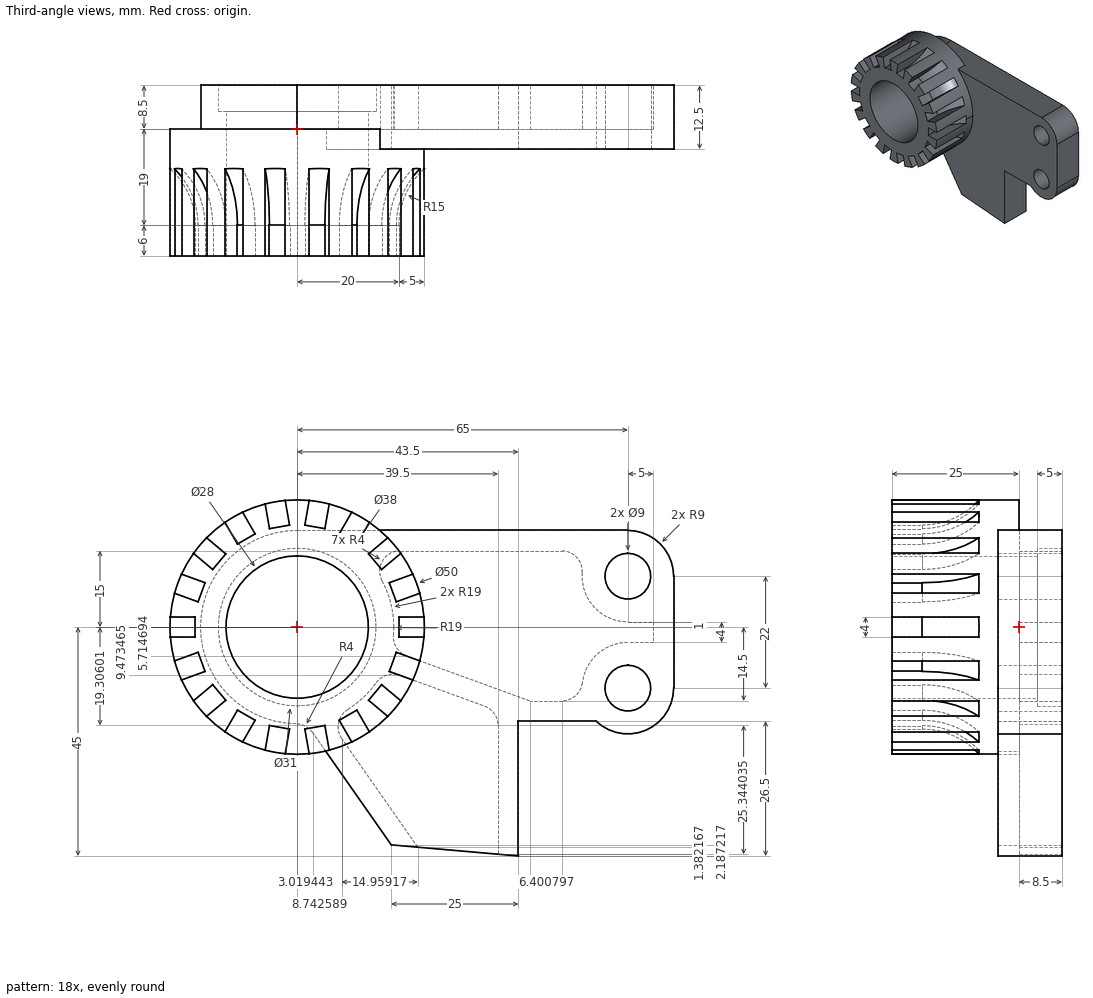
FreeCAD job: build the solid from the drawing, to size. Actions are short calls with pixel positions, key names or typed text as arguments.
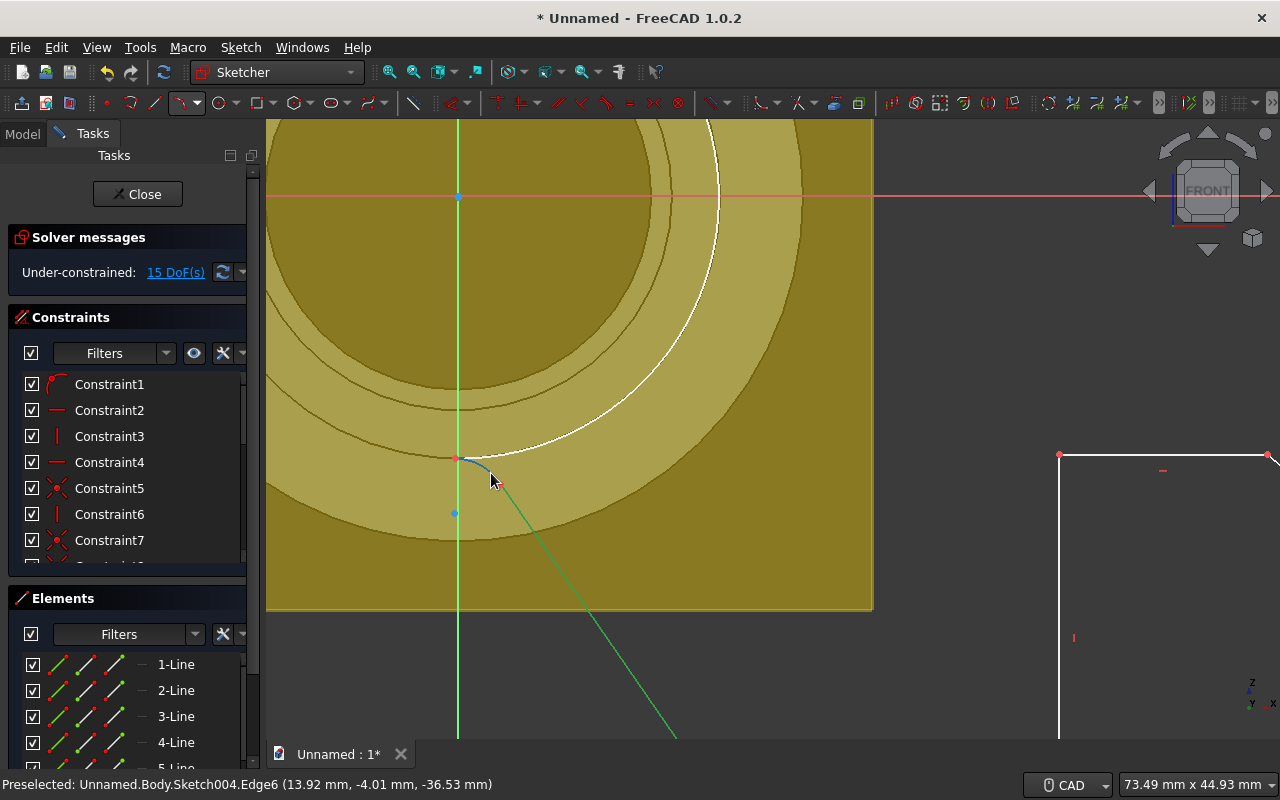
click(490, 472)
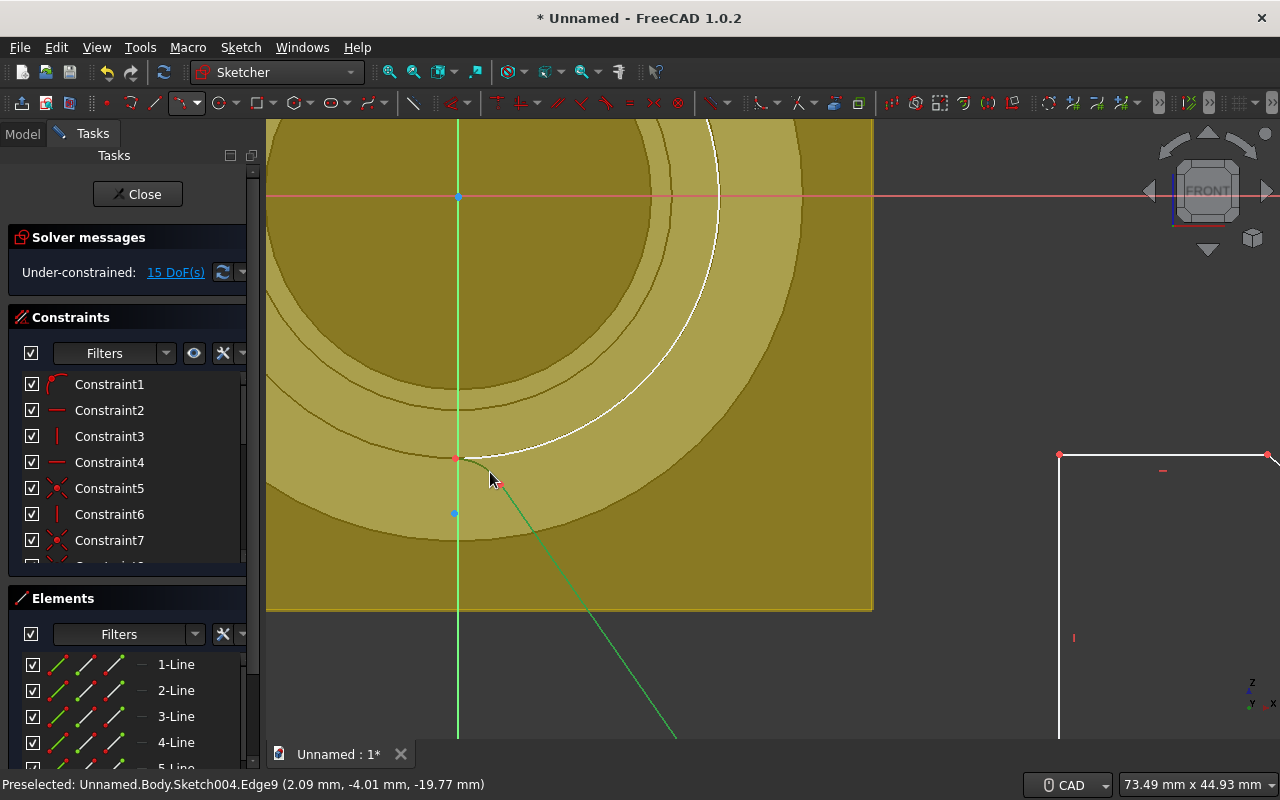
click(606, 104)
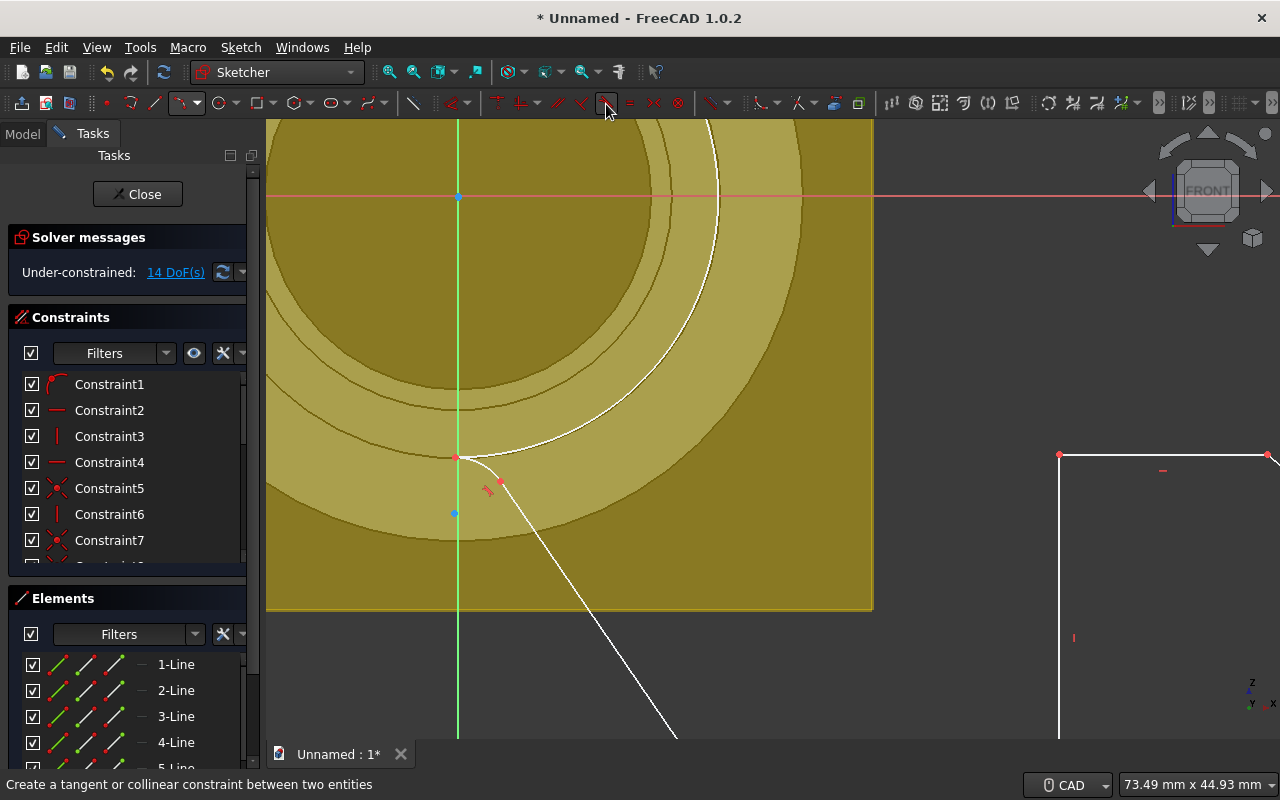
click(490, 470)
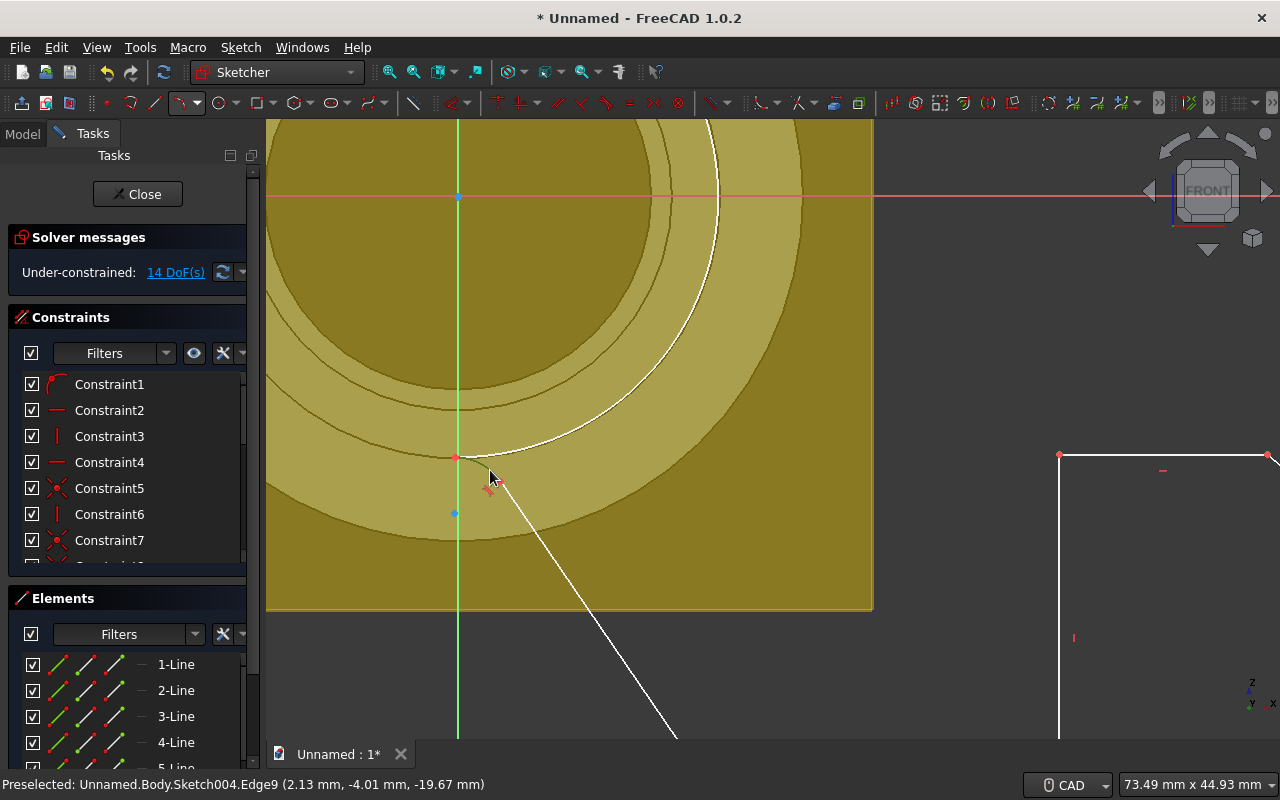
click(667, 352)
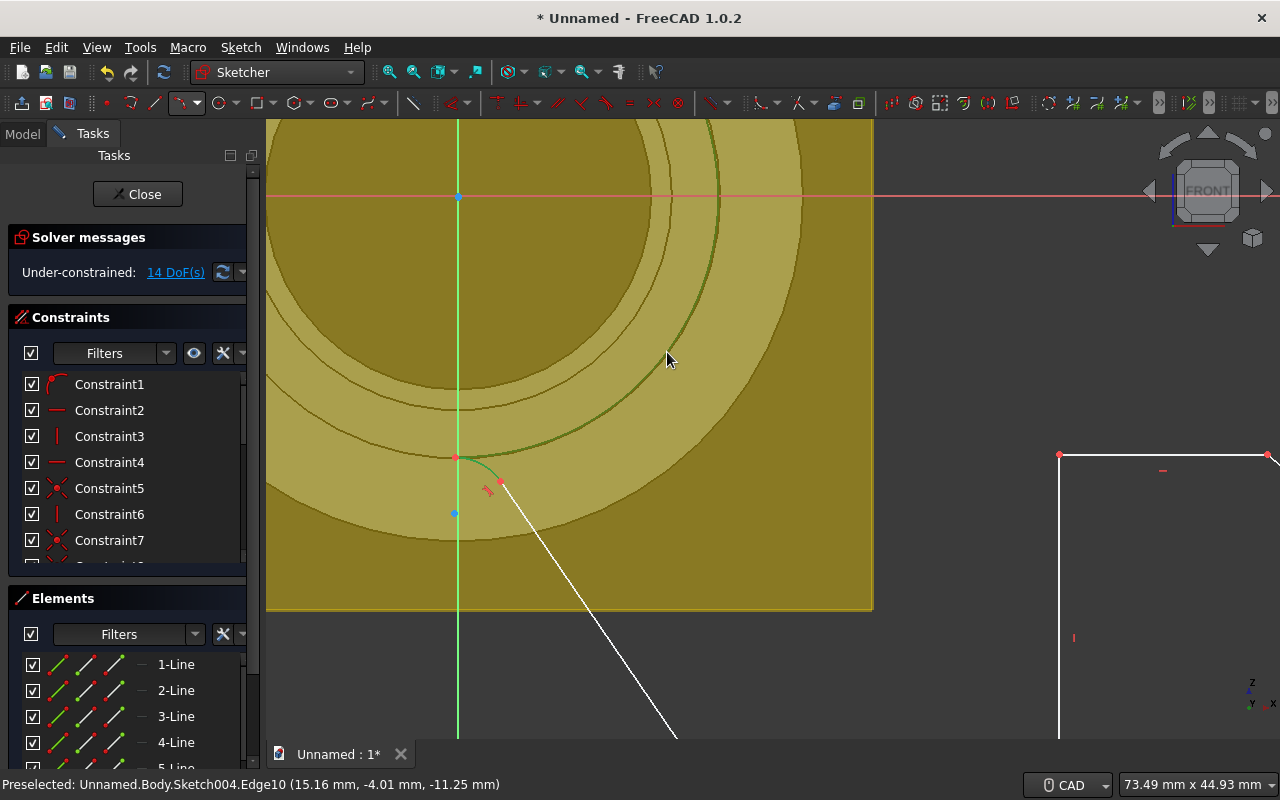
click(606, 104)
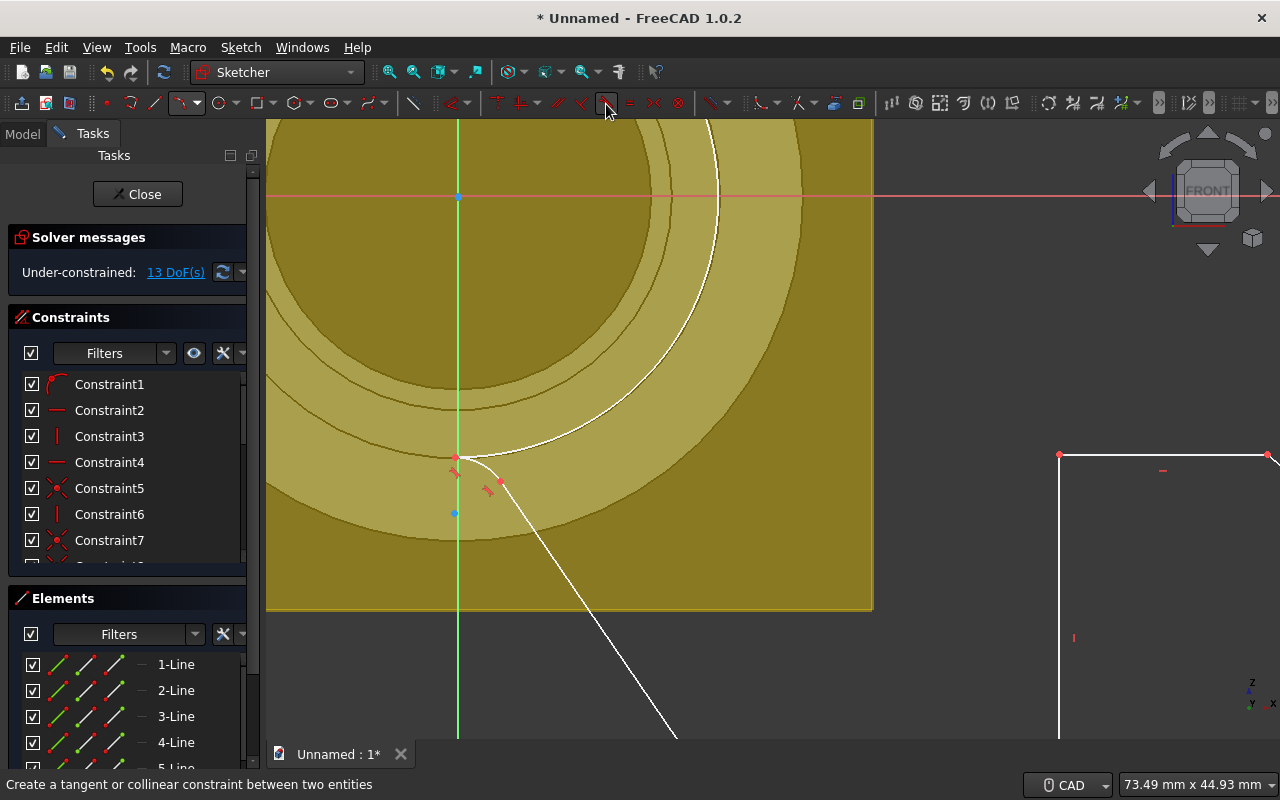
scroll(490, 472, down, 4)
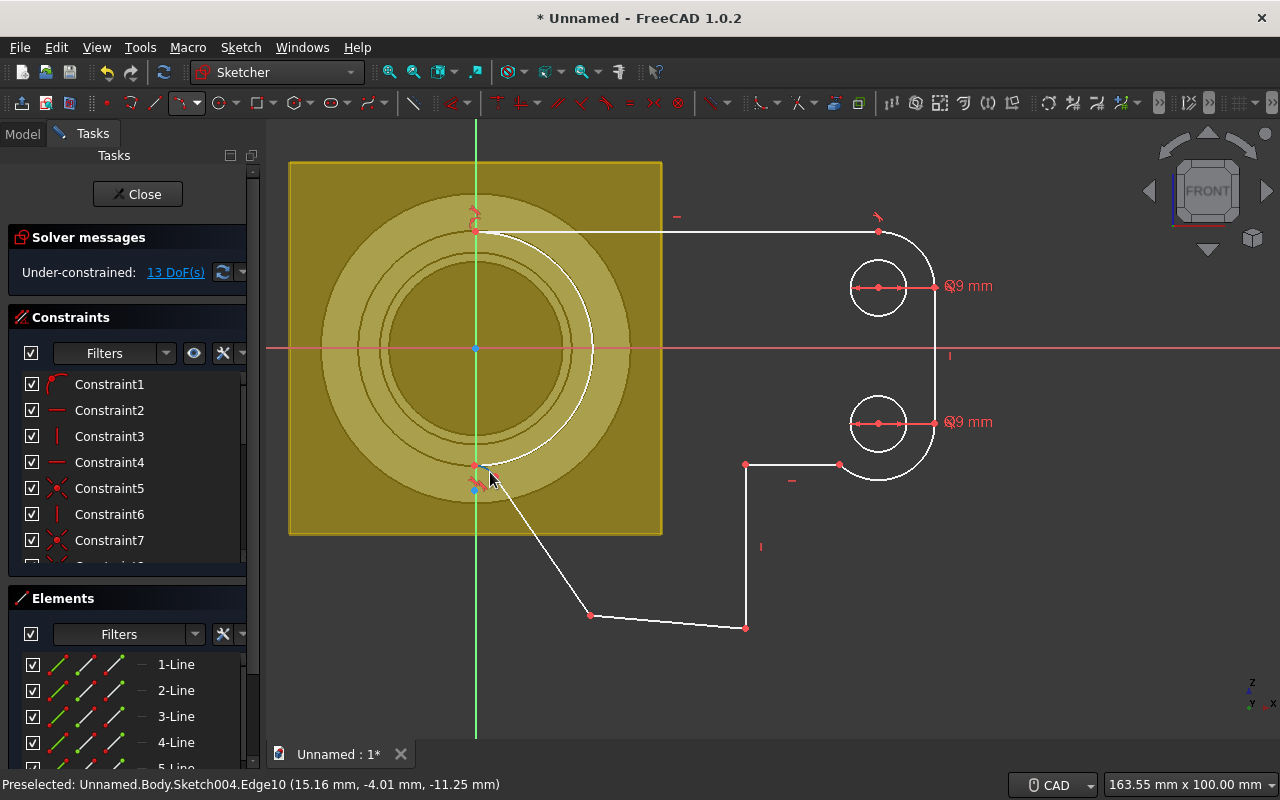
click(928, 263)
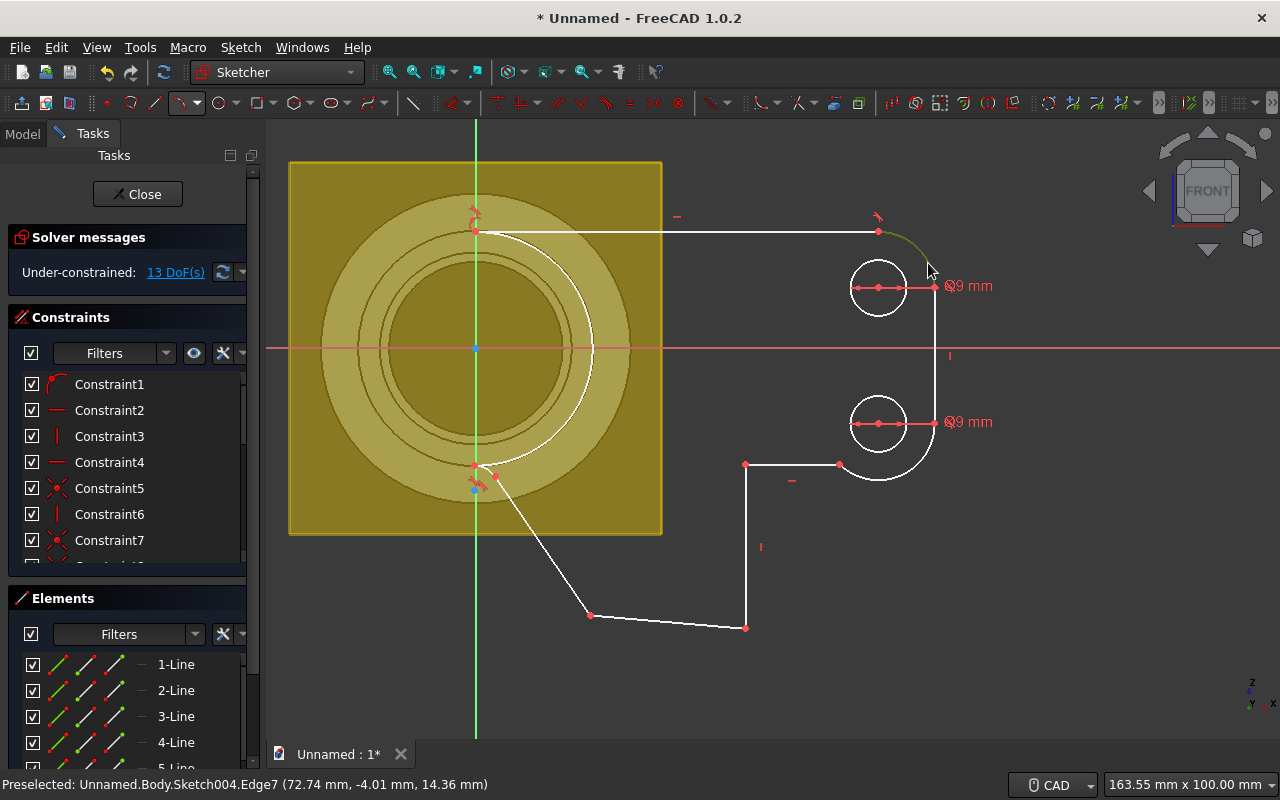
click(875, 480)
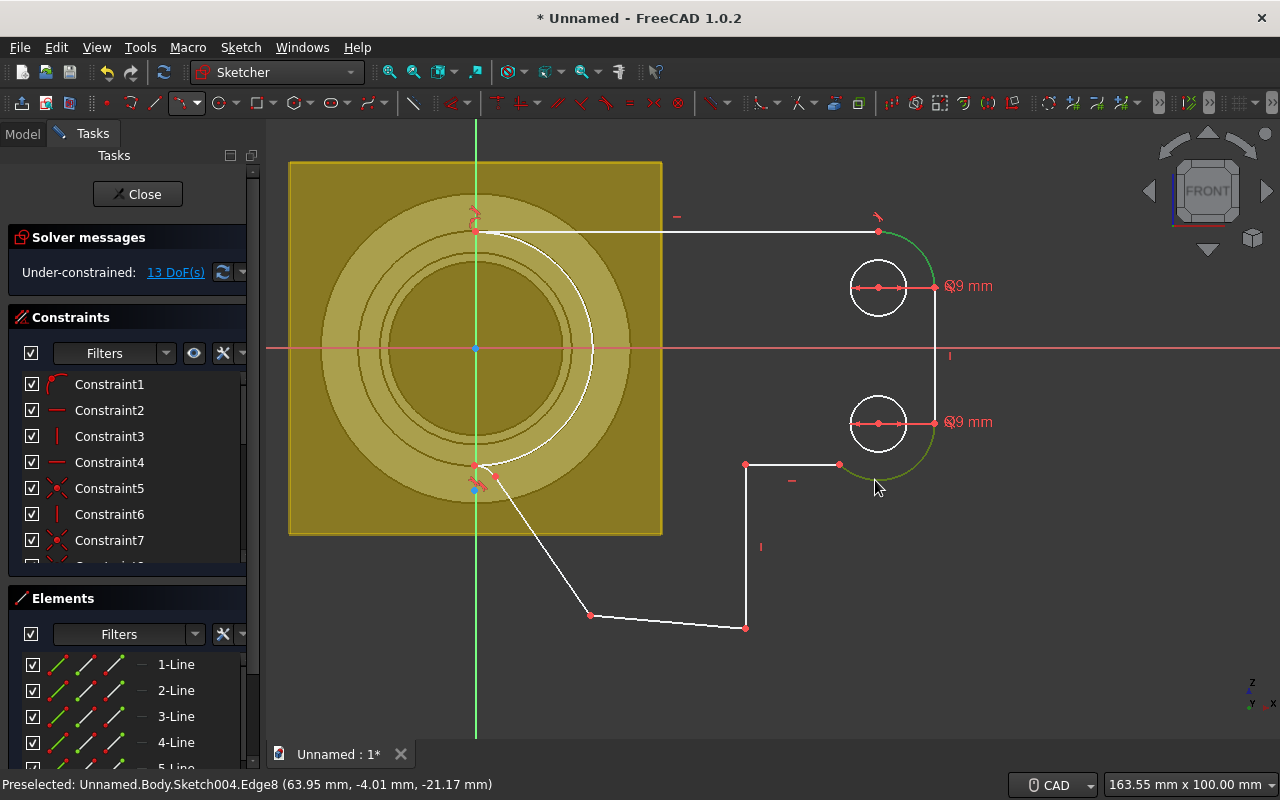
click(630, 104)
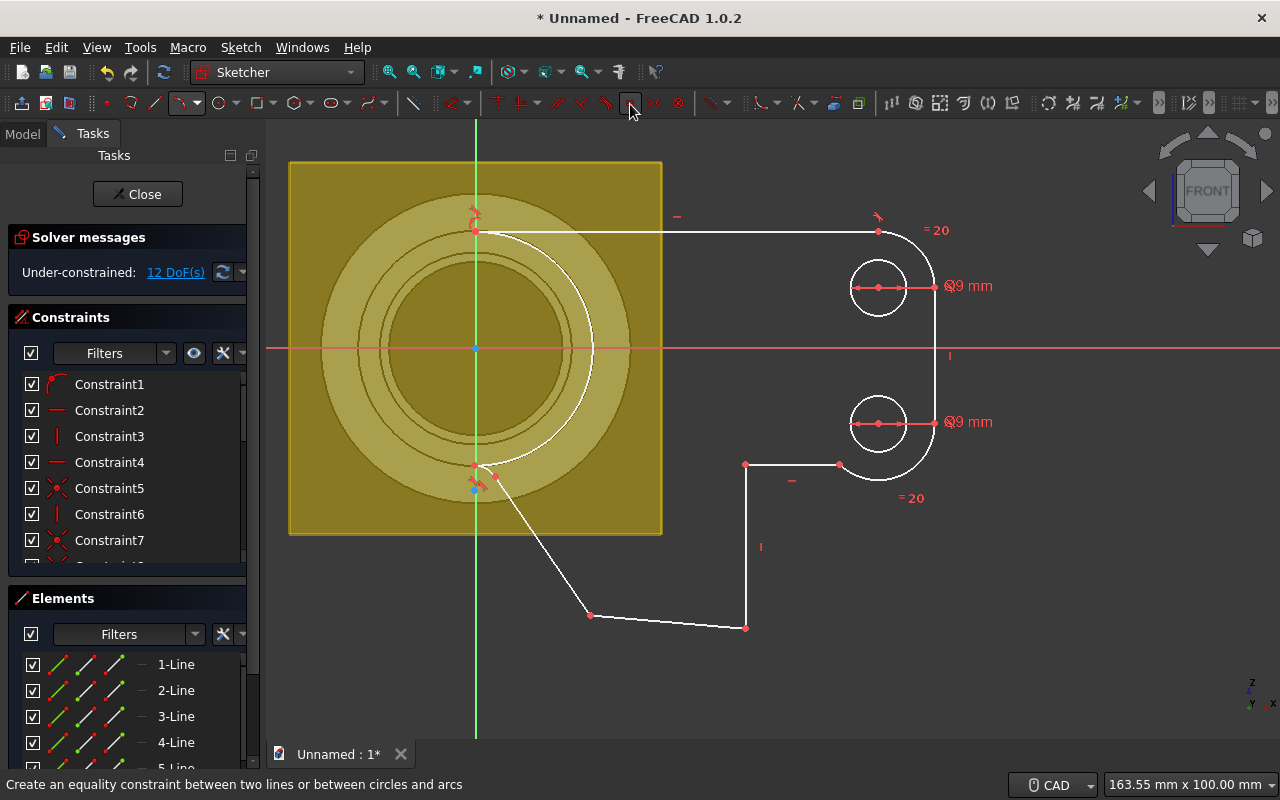
click(476, 349)